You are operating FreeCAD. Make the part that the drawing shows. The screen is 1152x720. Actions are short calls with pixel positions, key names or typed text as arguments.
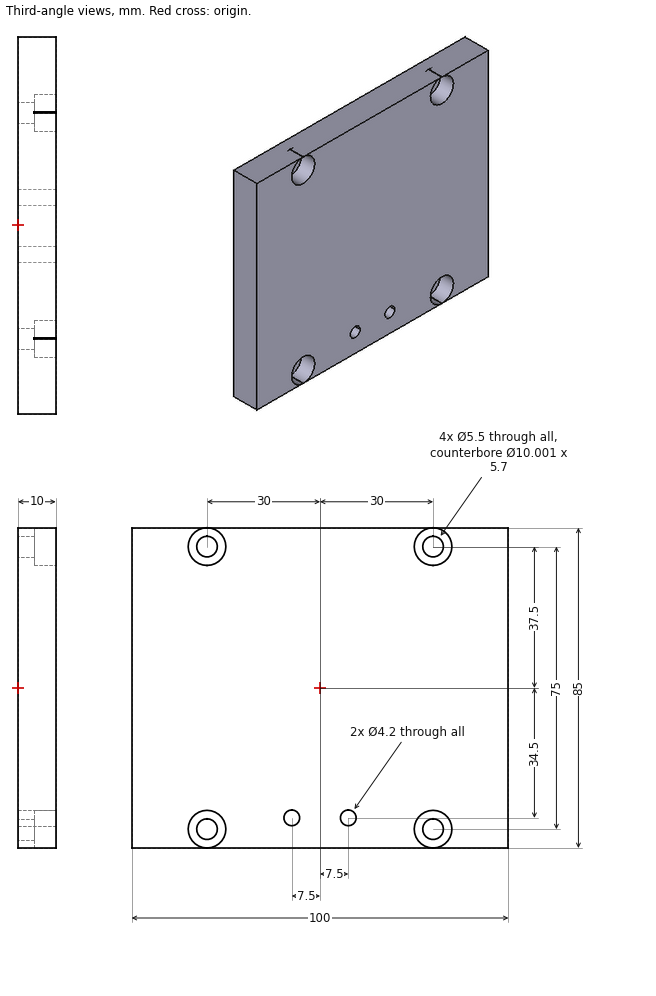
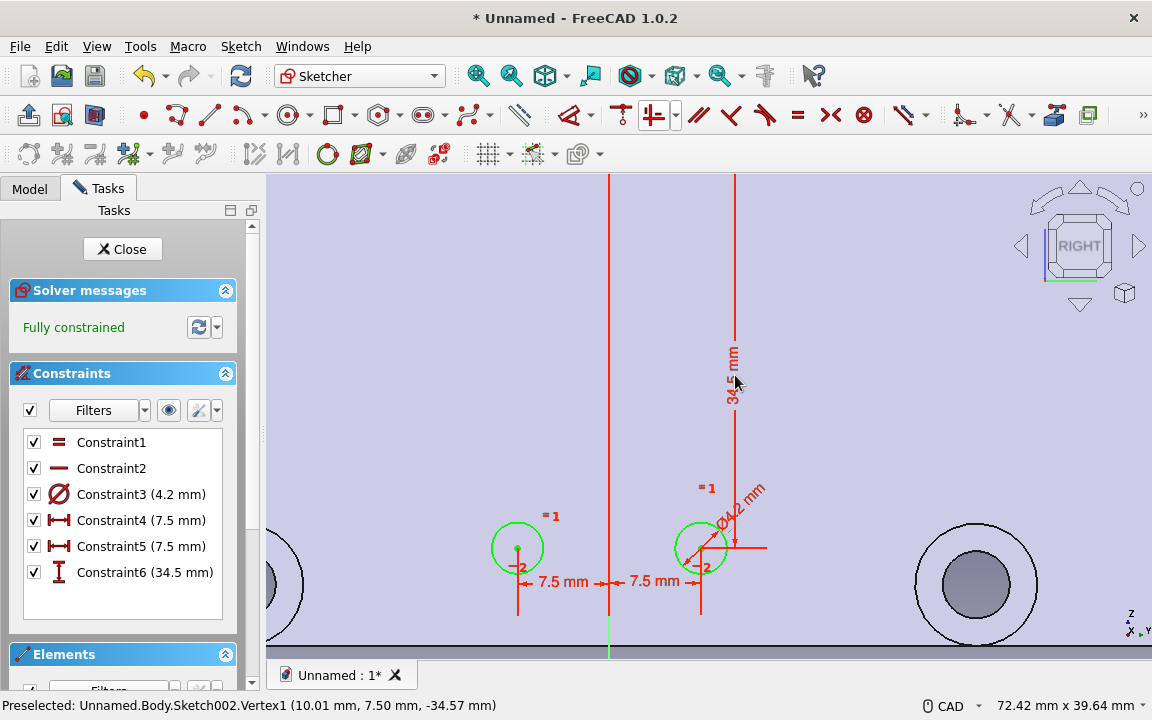
click(123, 249)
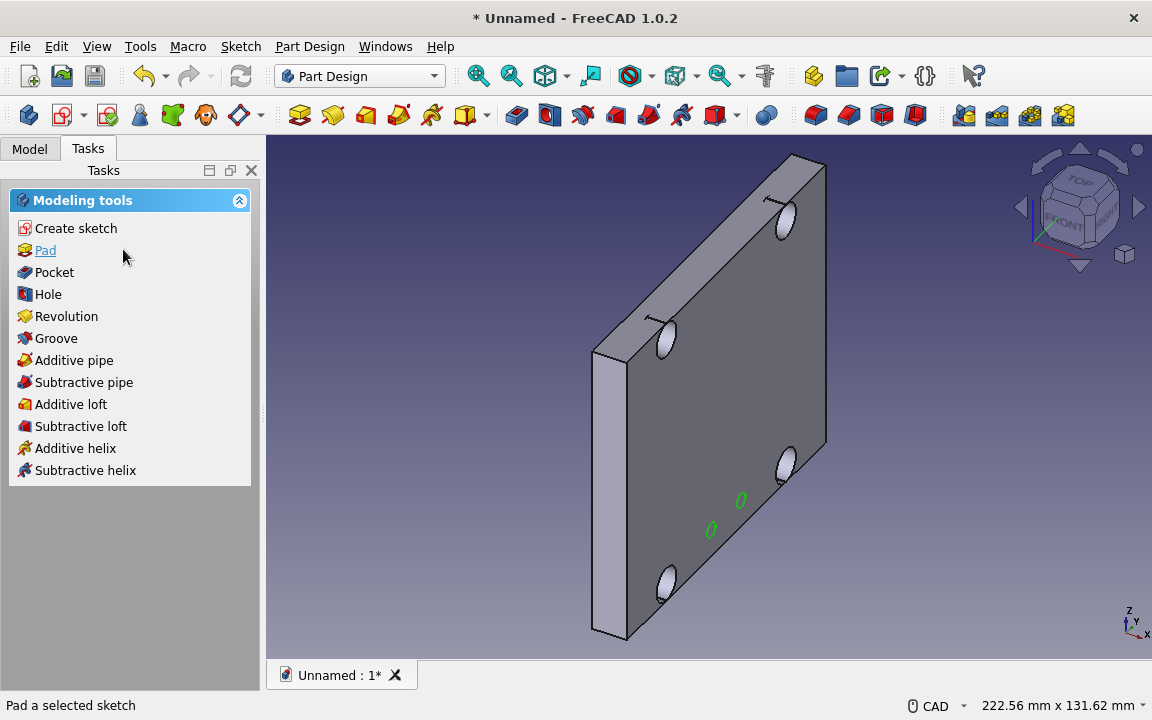
click(550, 116)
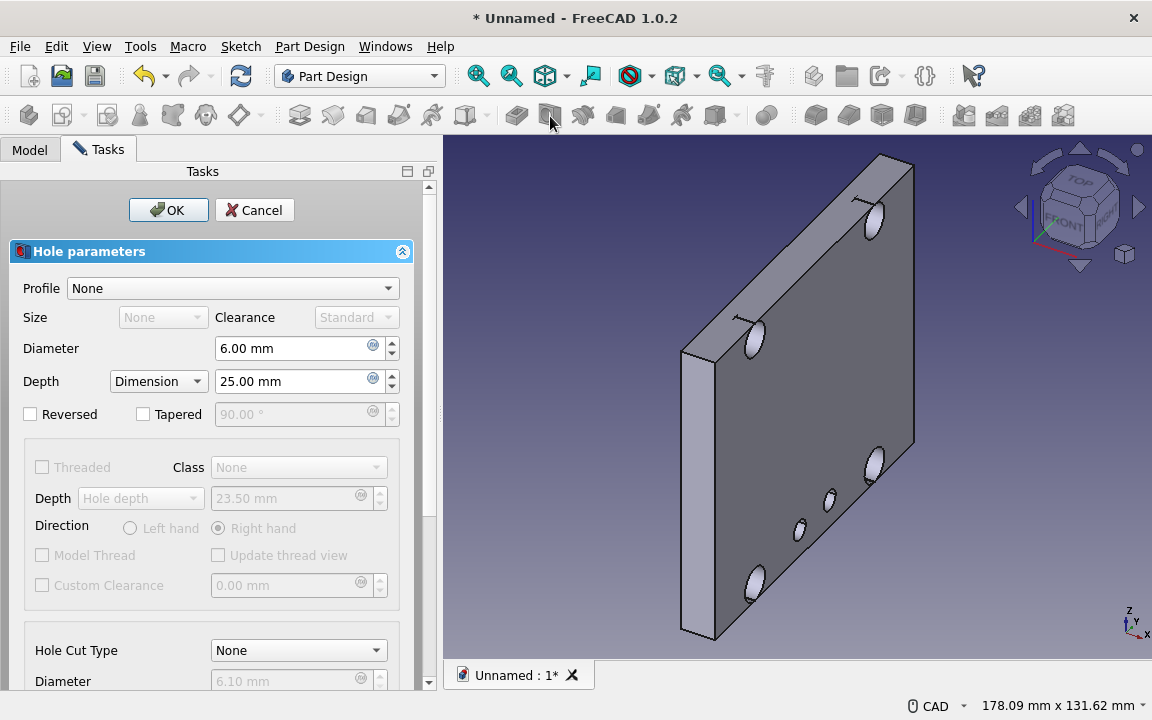
triple_click(300, 348)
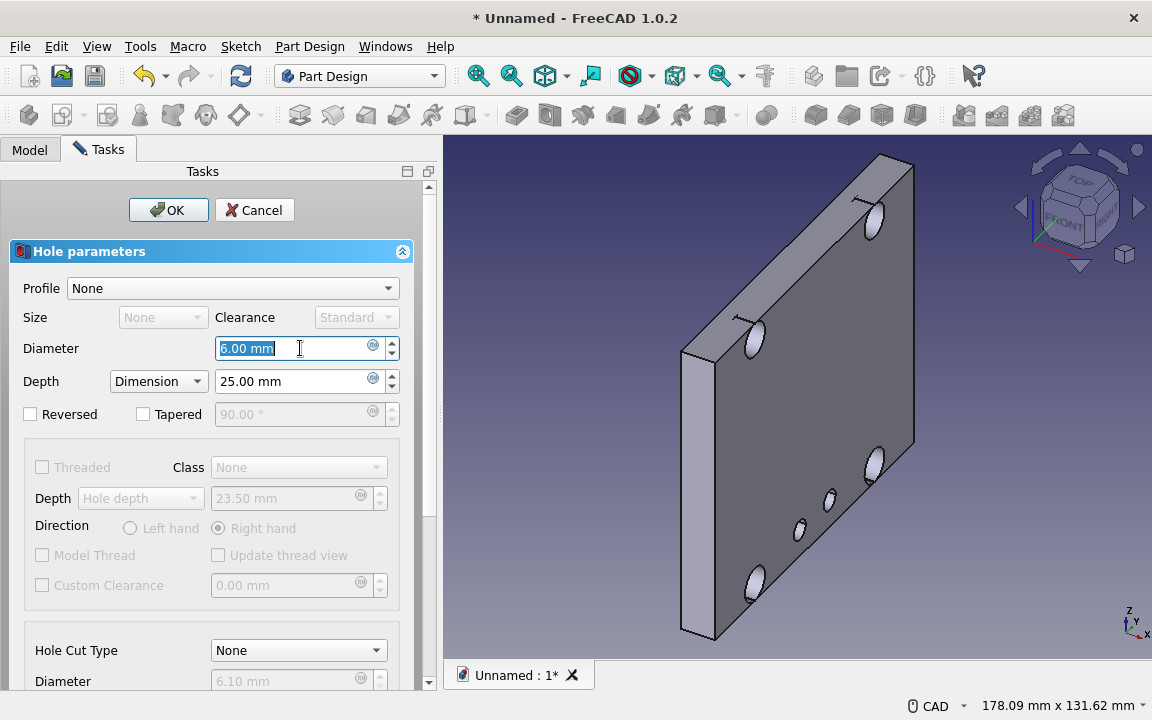
text(4.2)
key(Tab)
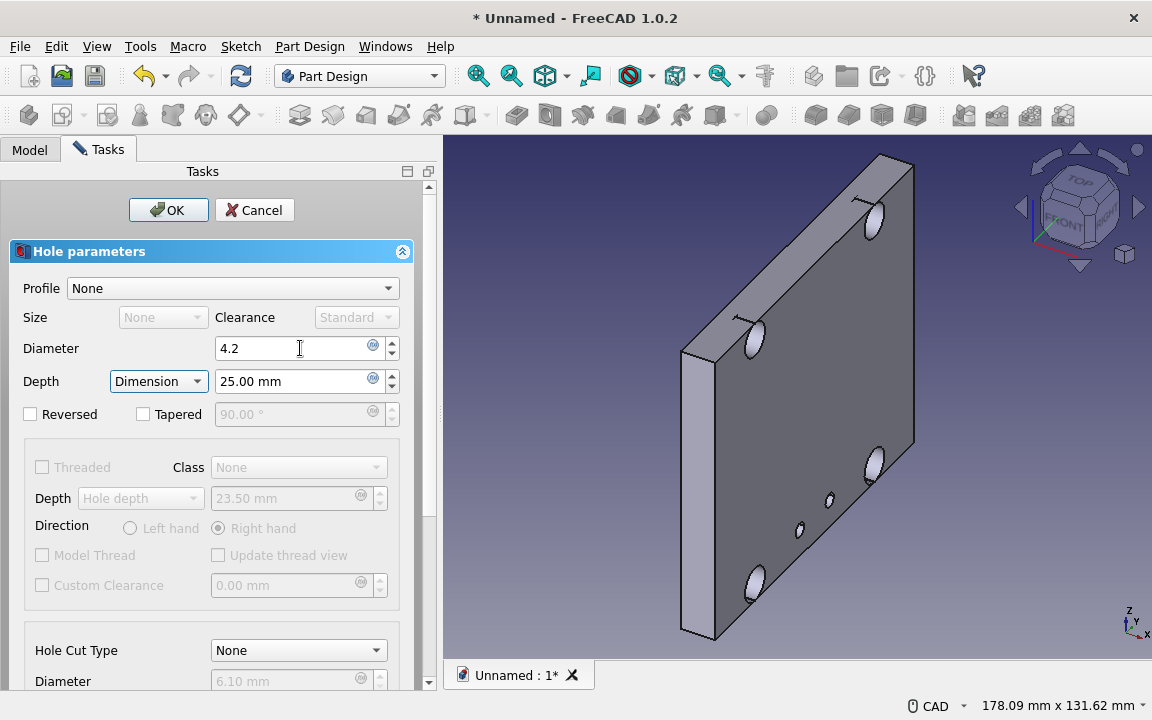
click(160, 382)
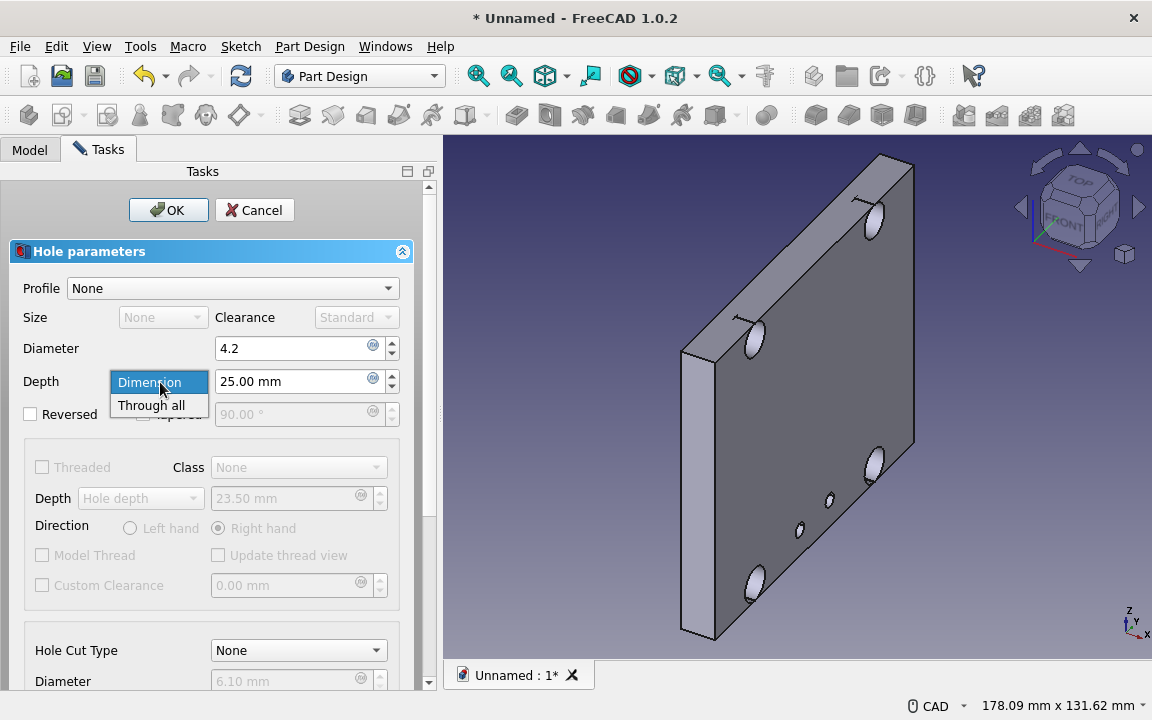
click(158, 406)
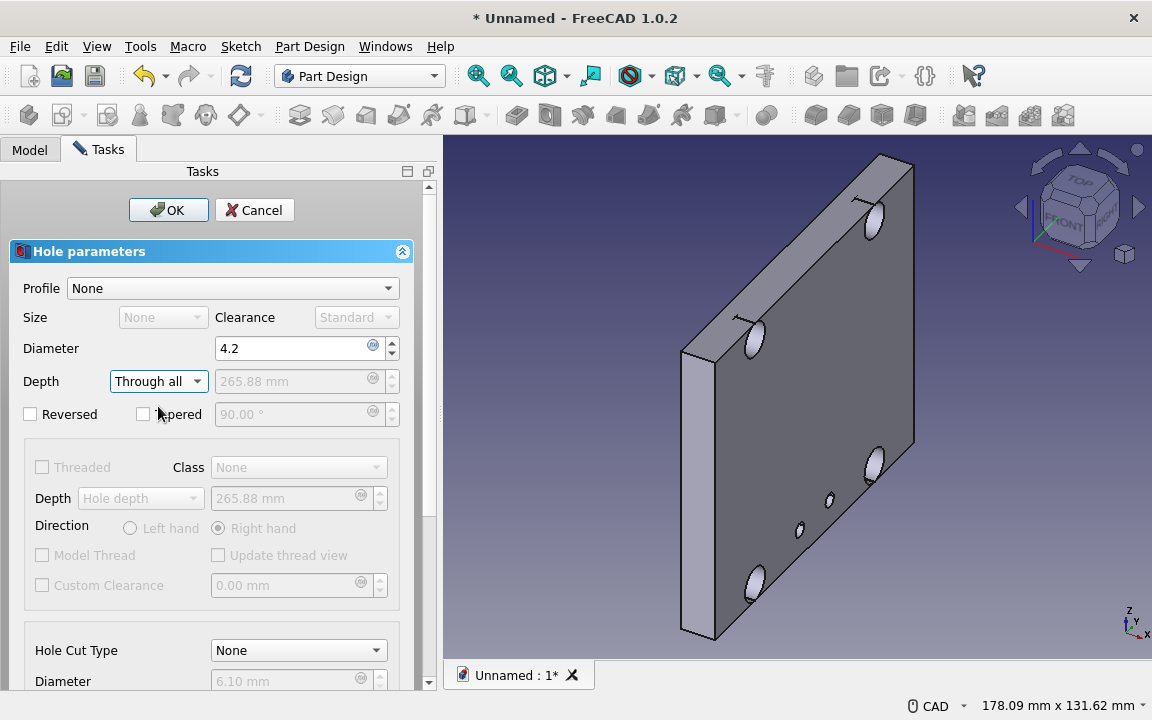
click(169, 210)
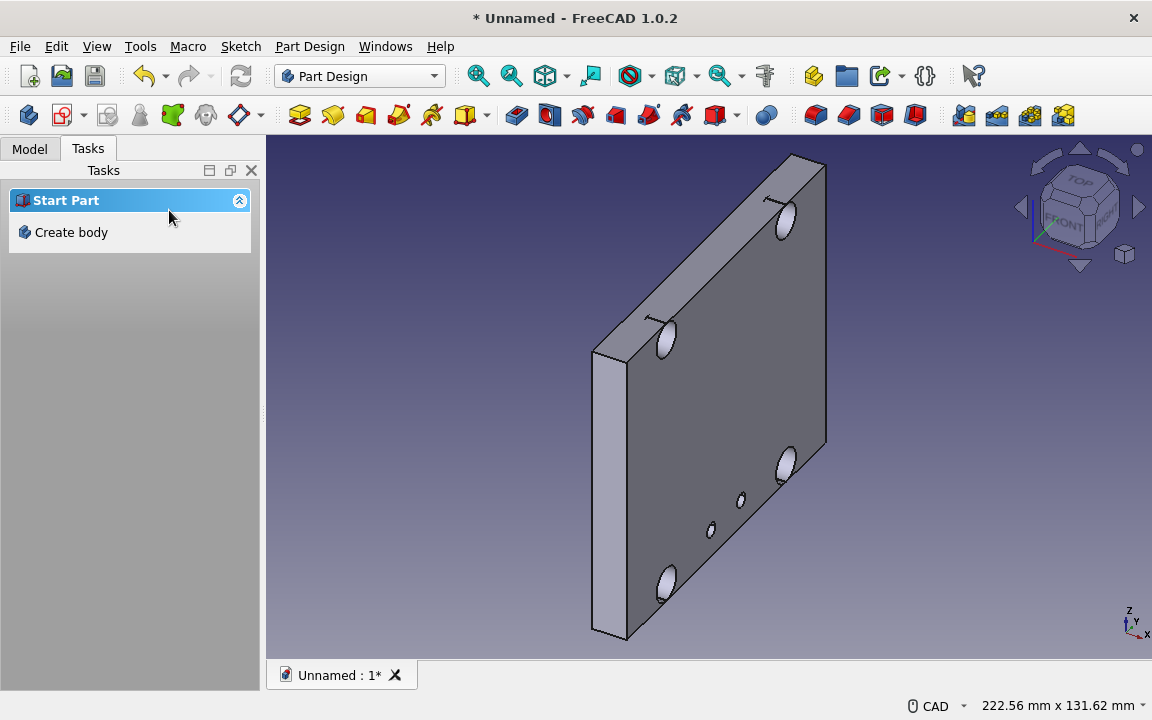
key(0)